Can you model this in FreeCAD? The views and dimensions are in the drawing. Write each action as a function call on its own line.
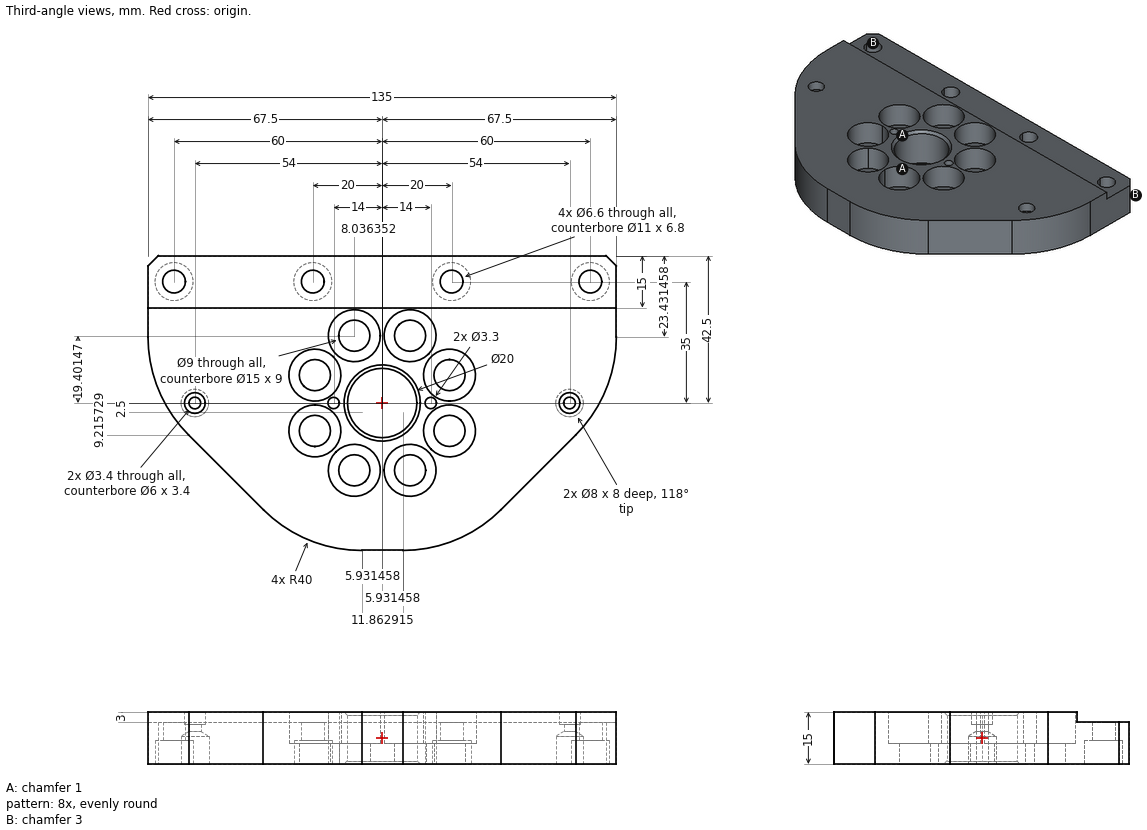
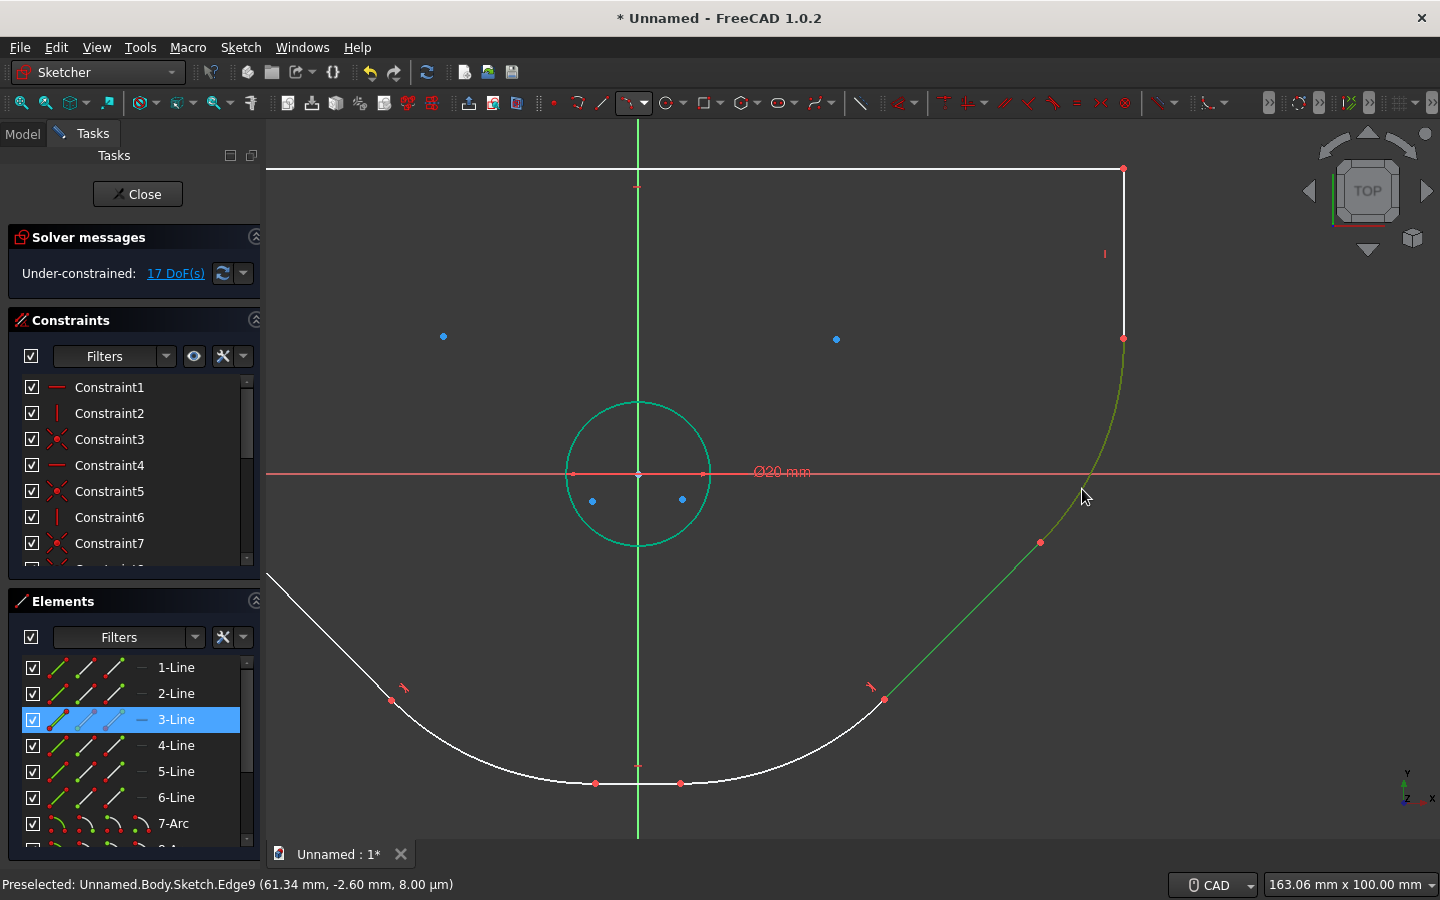
click(1054, 104)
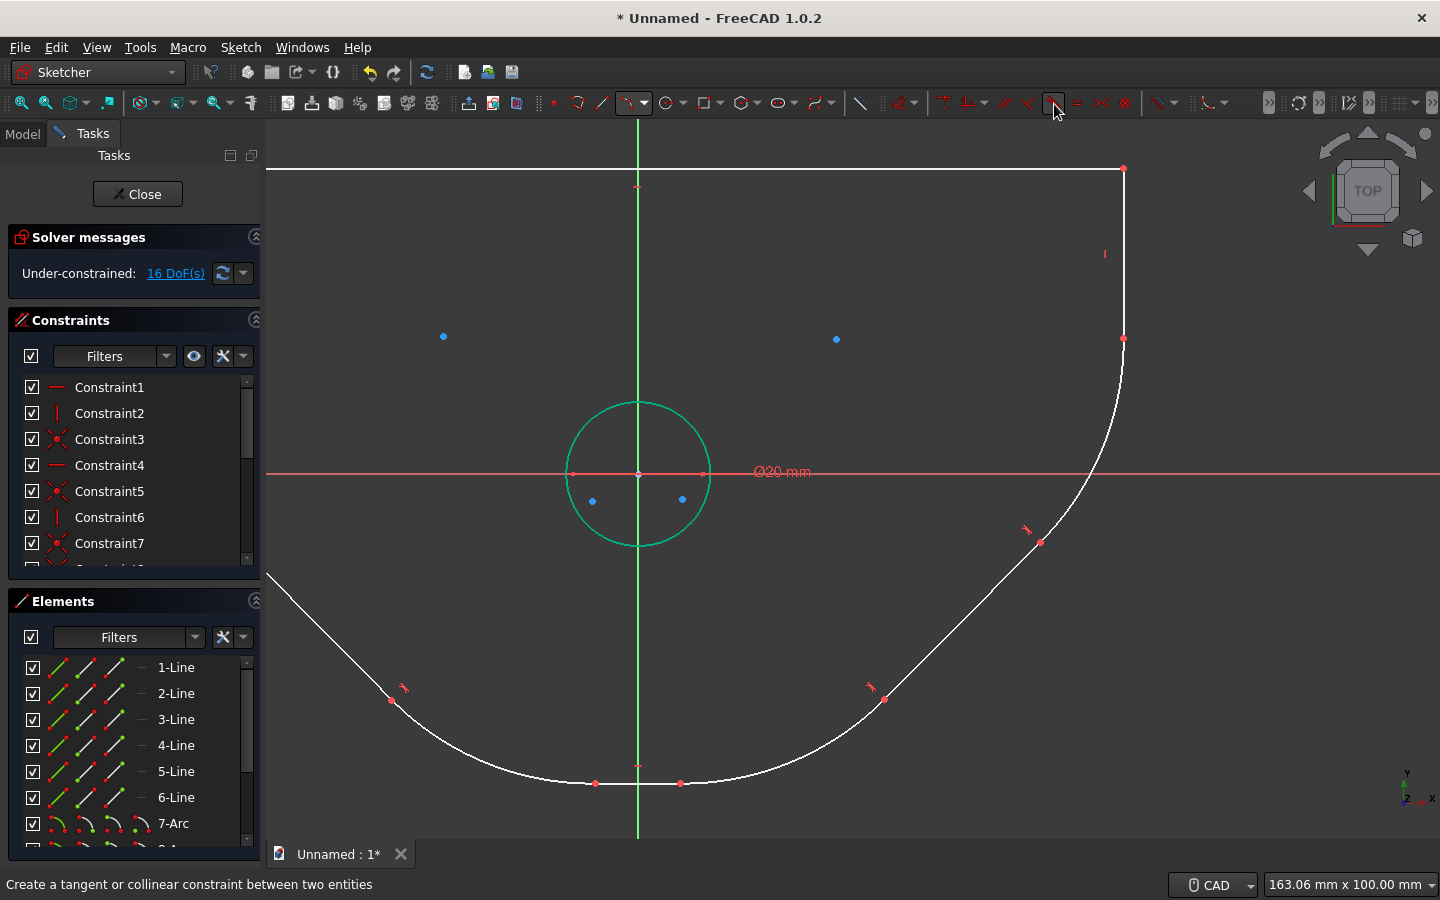
click(445, 742)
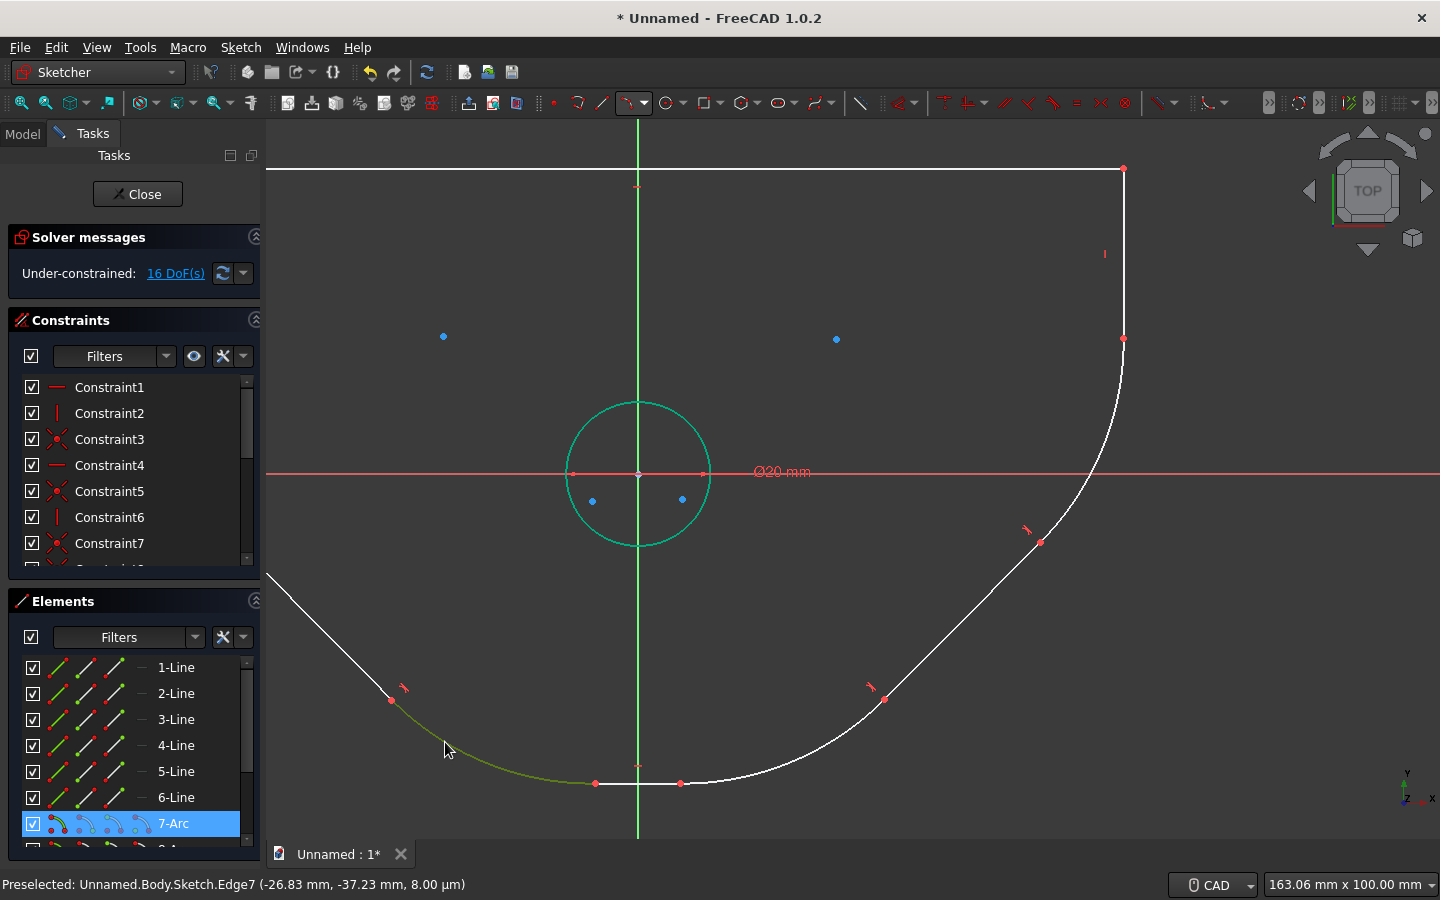
click(748, 776)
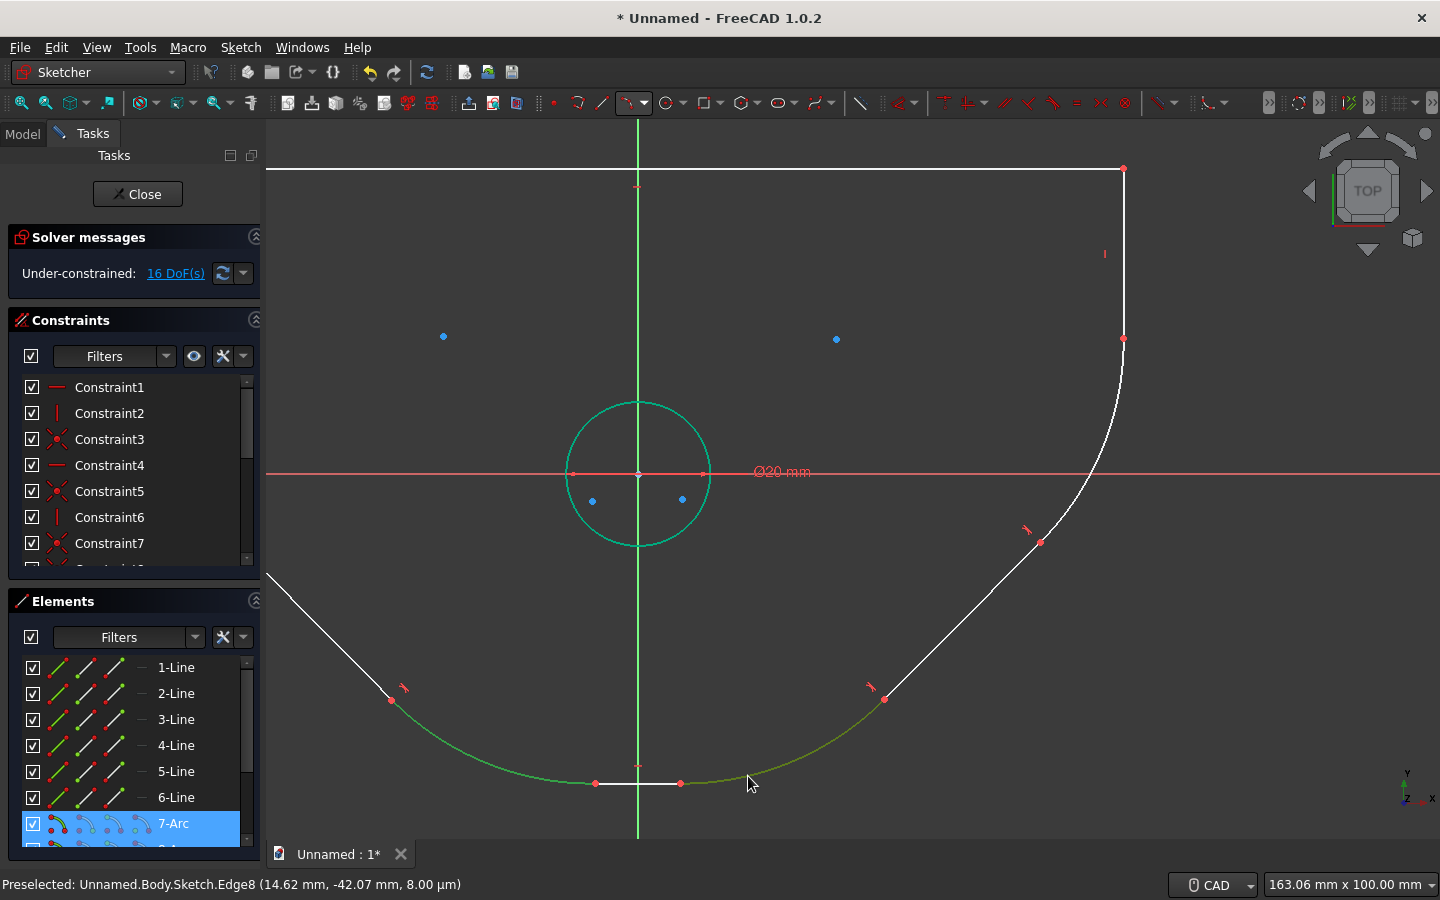
click(1082, 489)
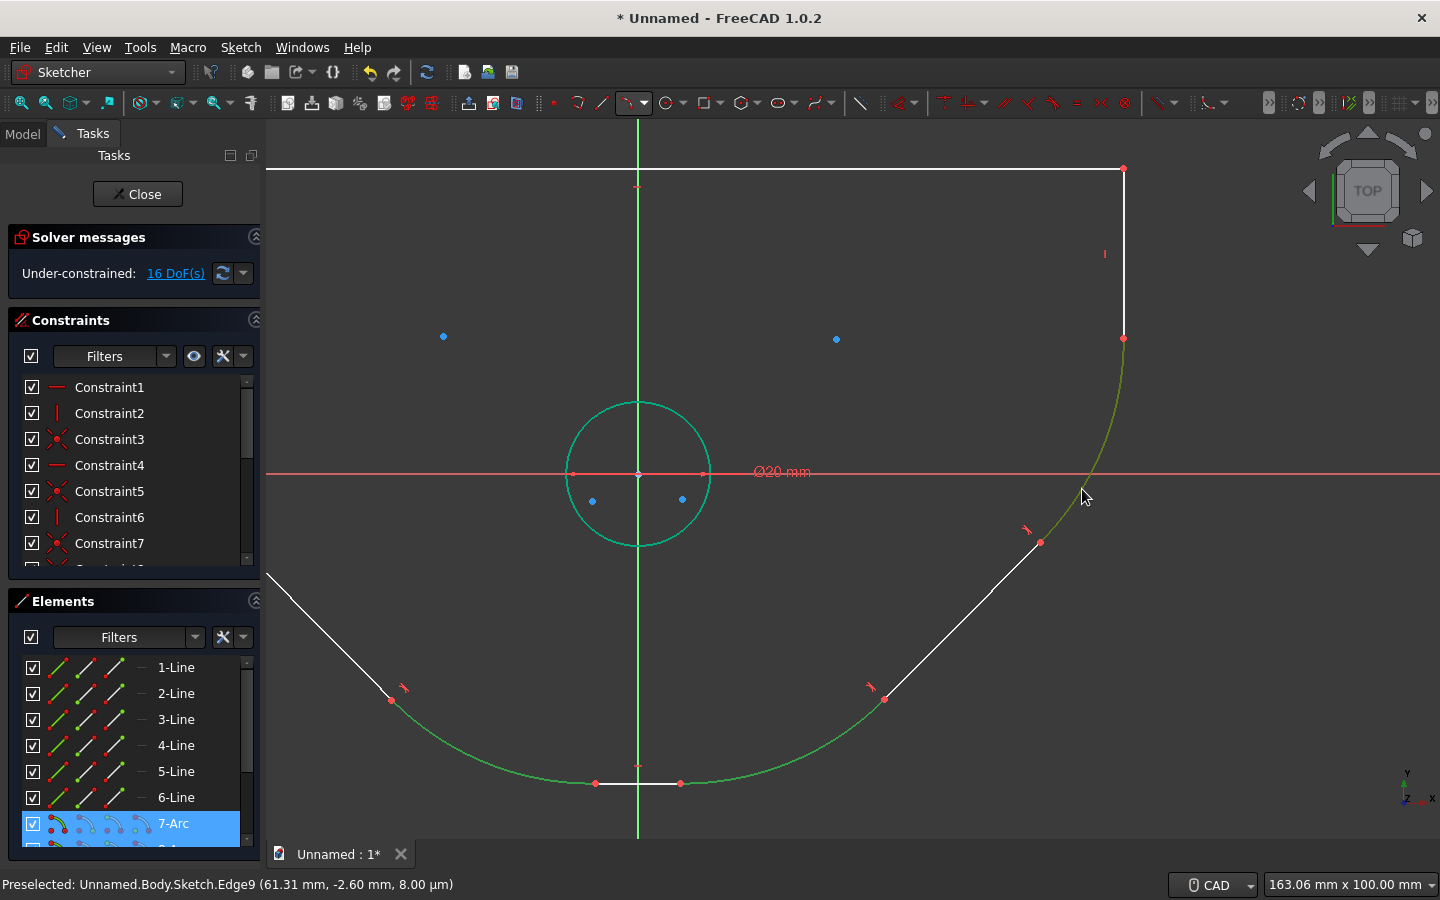
scroll(1082, 489, down, 2)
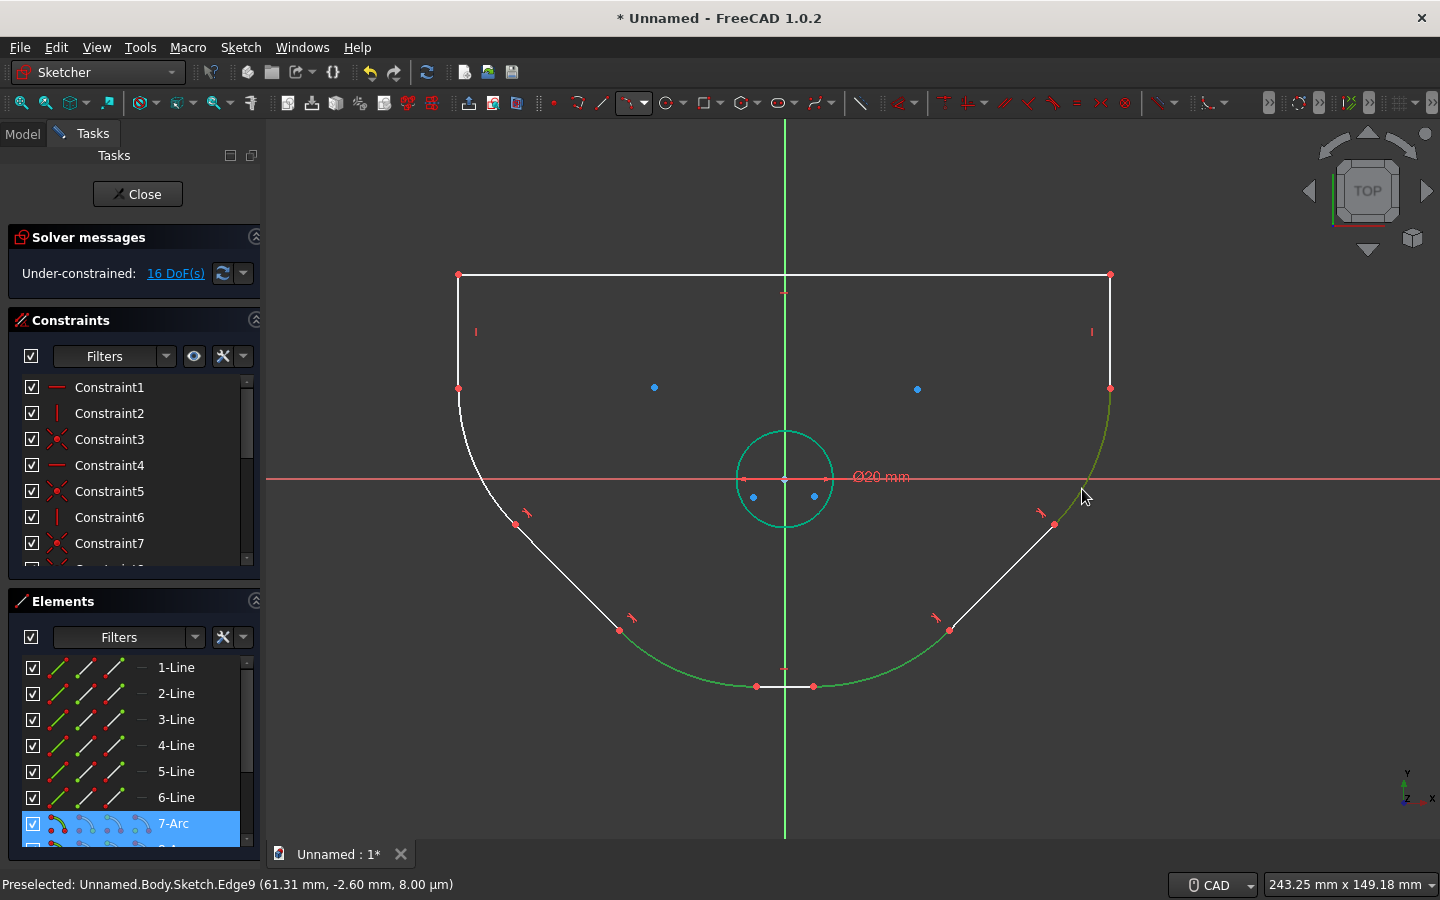
click(464, 433)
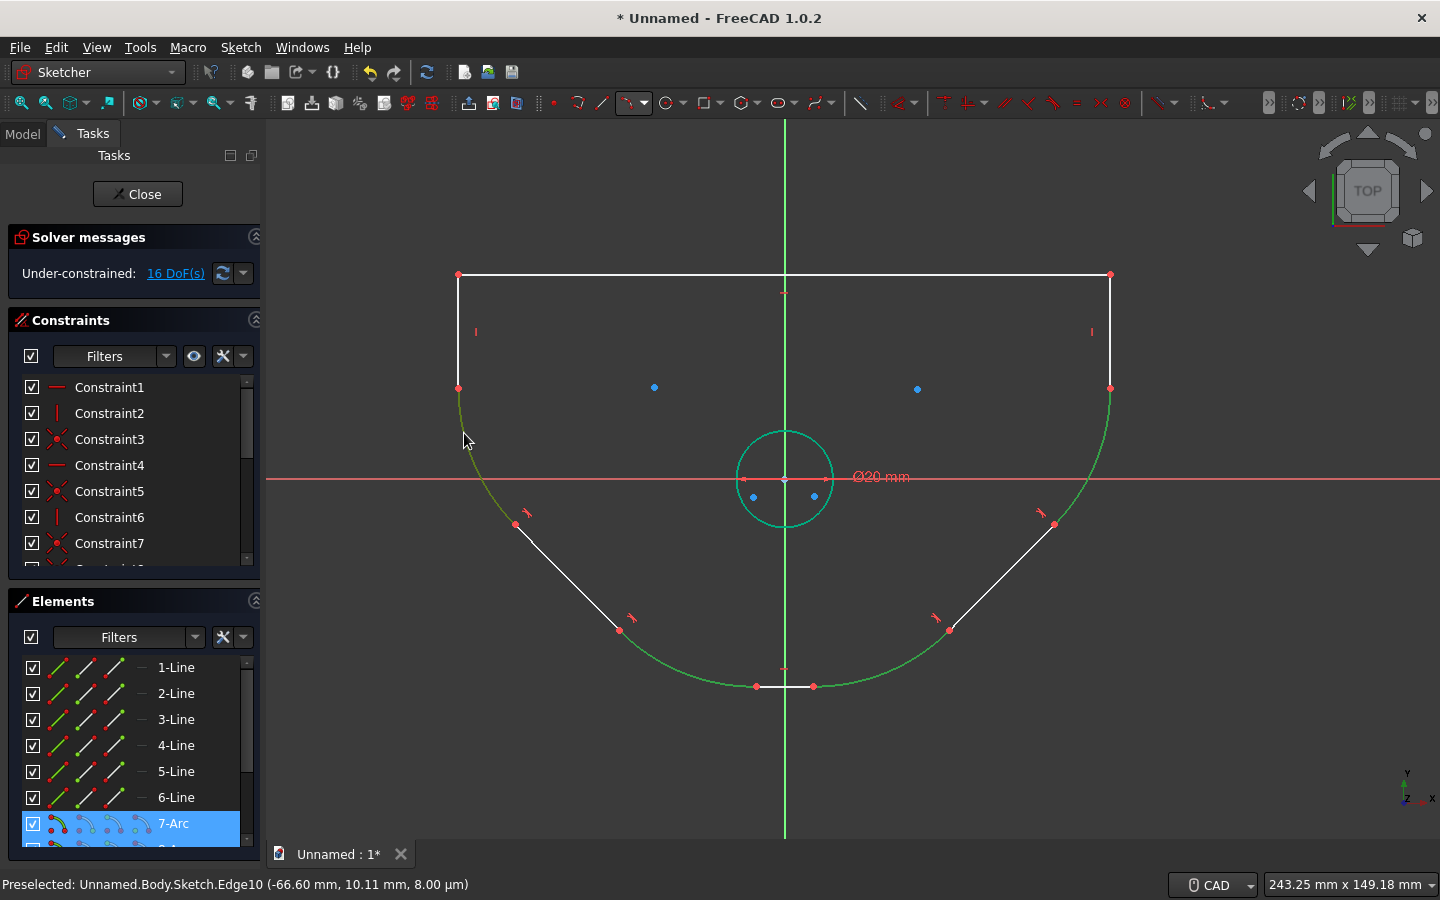
click(1078, 104)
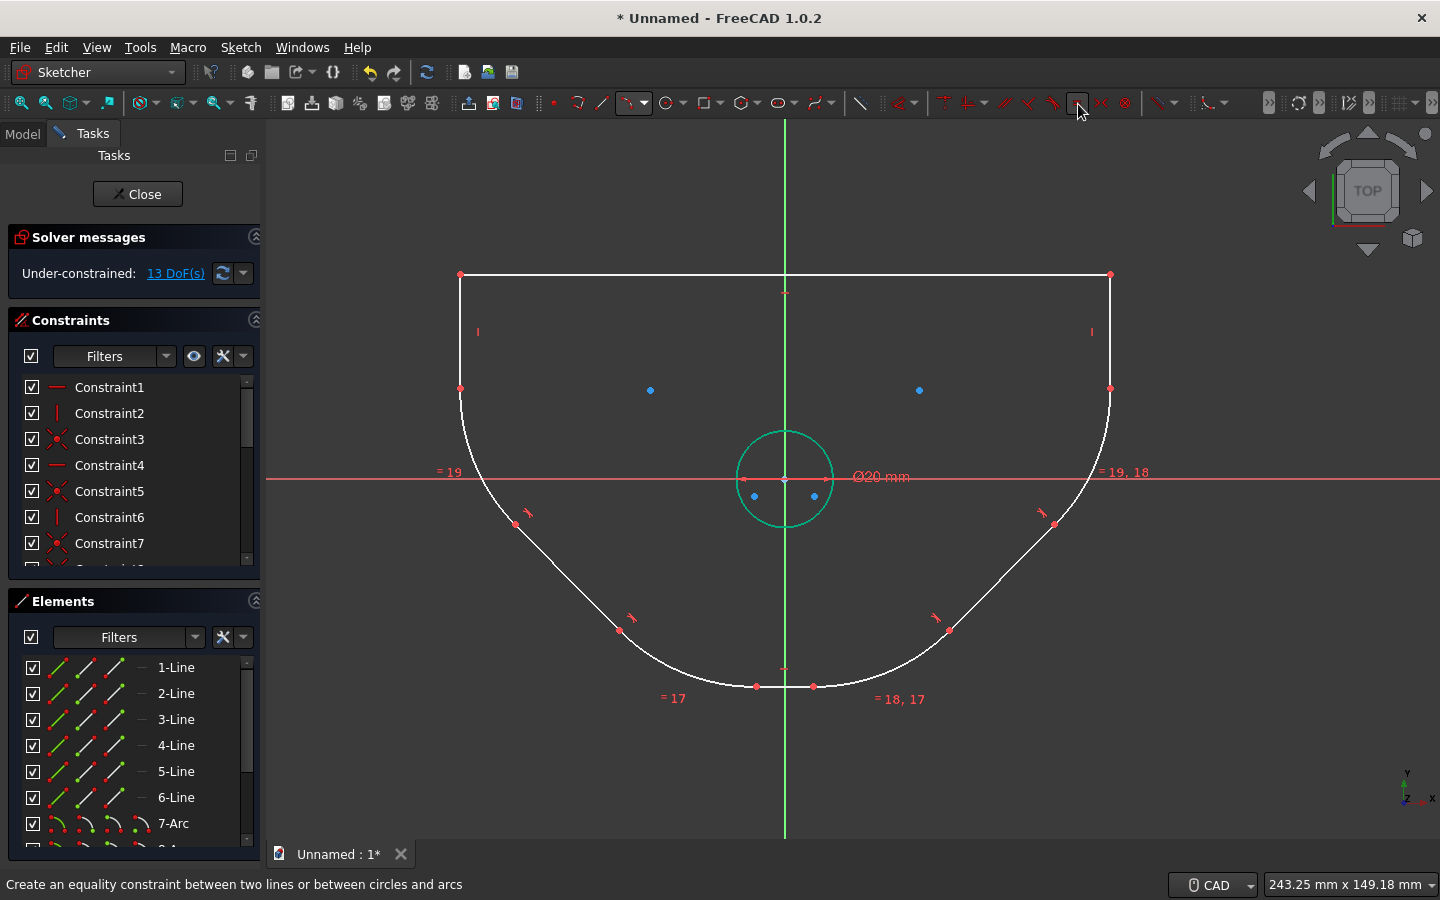
click(898, 104)